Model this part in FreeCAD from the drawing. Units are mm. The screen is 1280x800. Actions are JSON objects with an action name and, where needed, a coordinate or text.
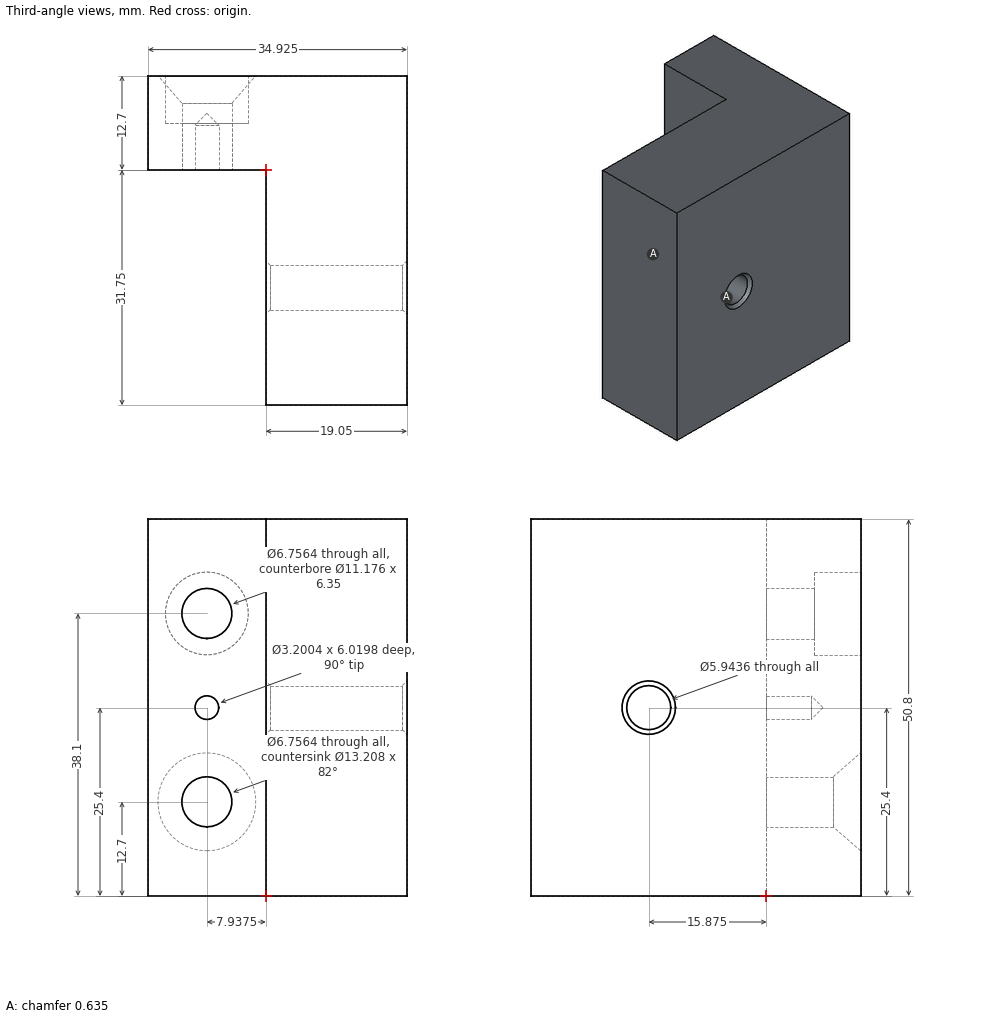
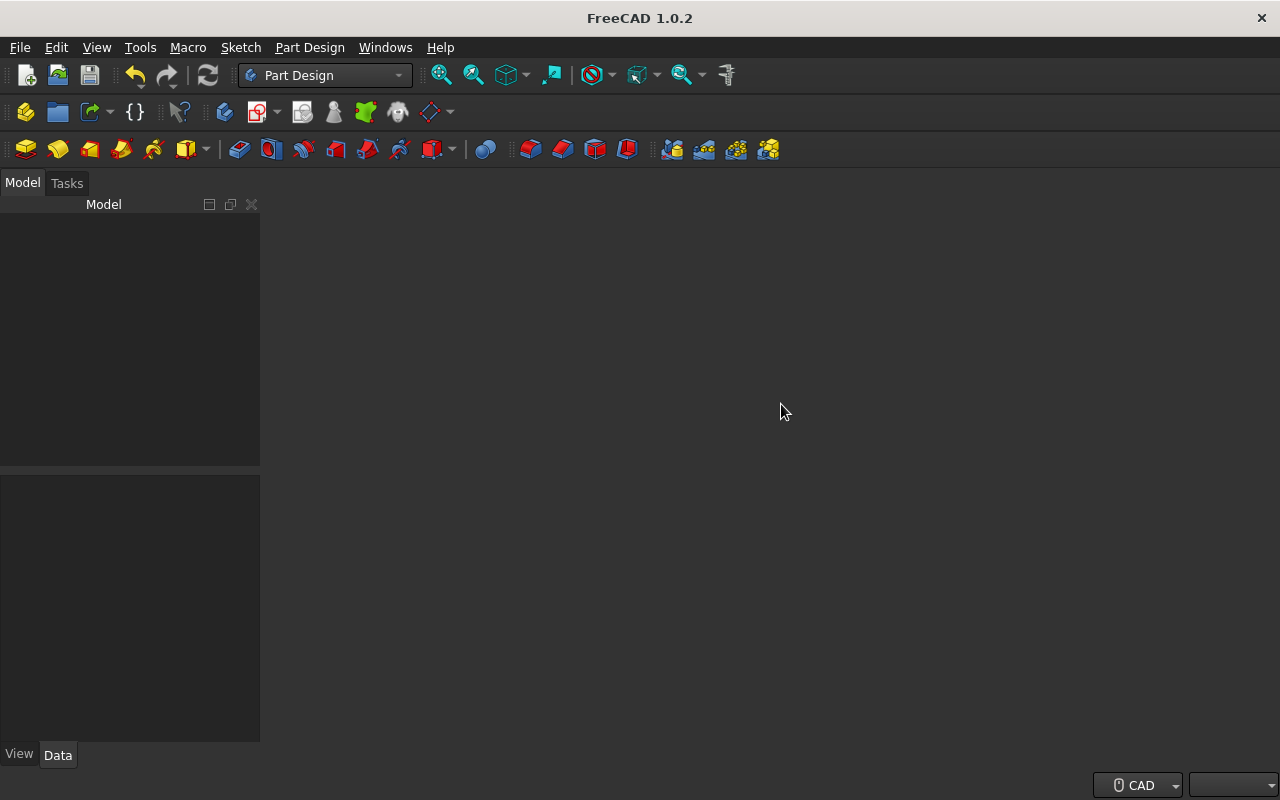
{"action": "left_click", "coordinate": [26, 76]}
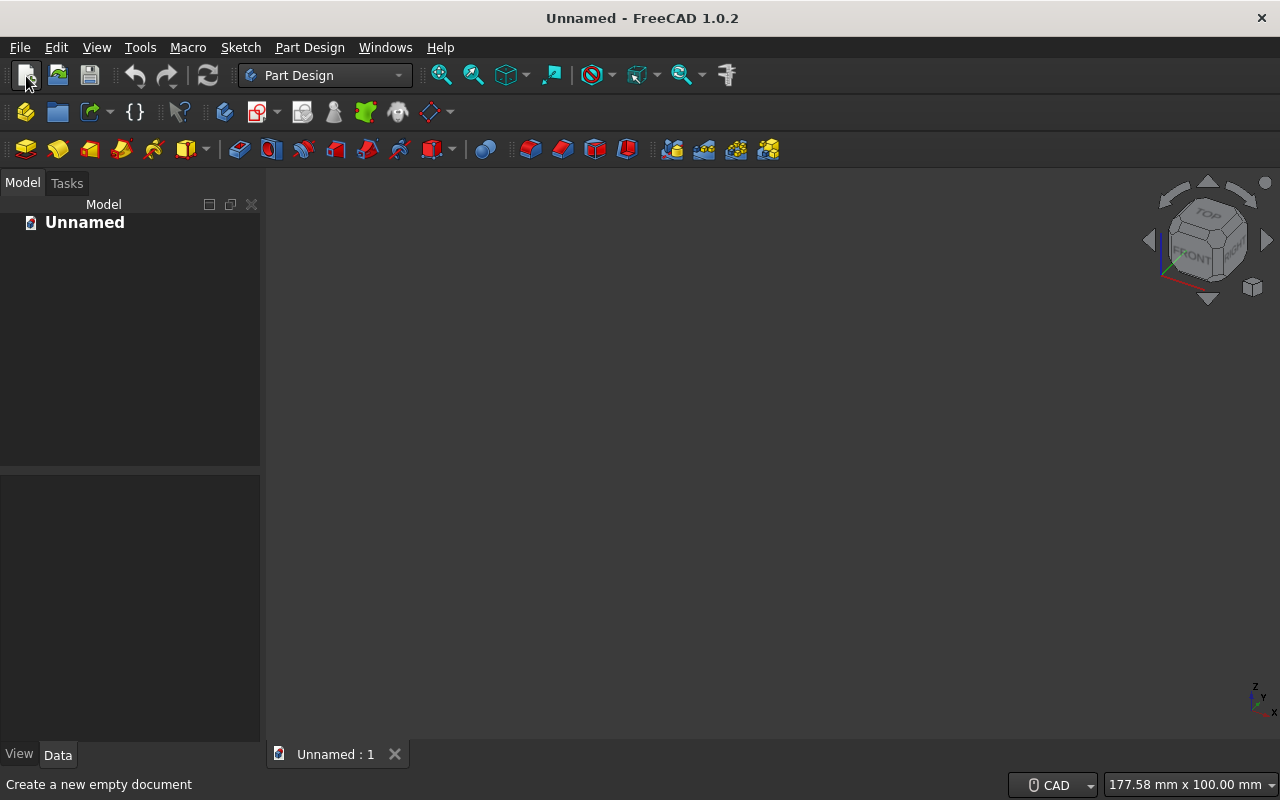
{"action": "left_click", "coordinate": [258, 112]}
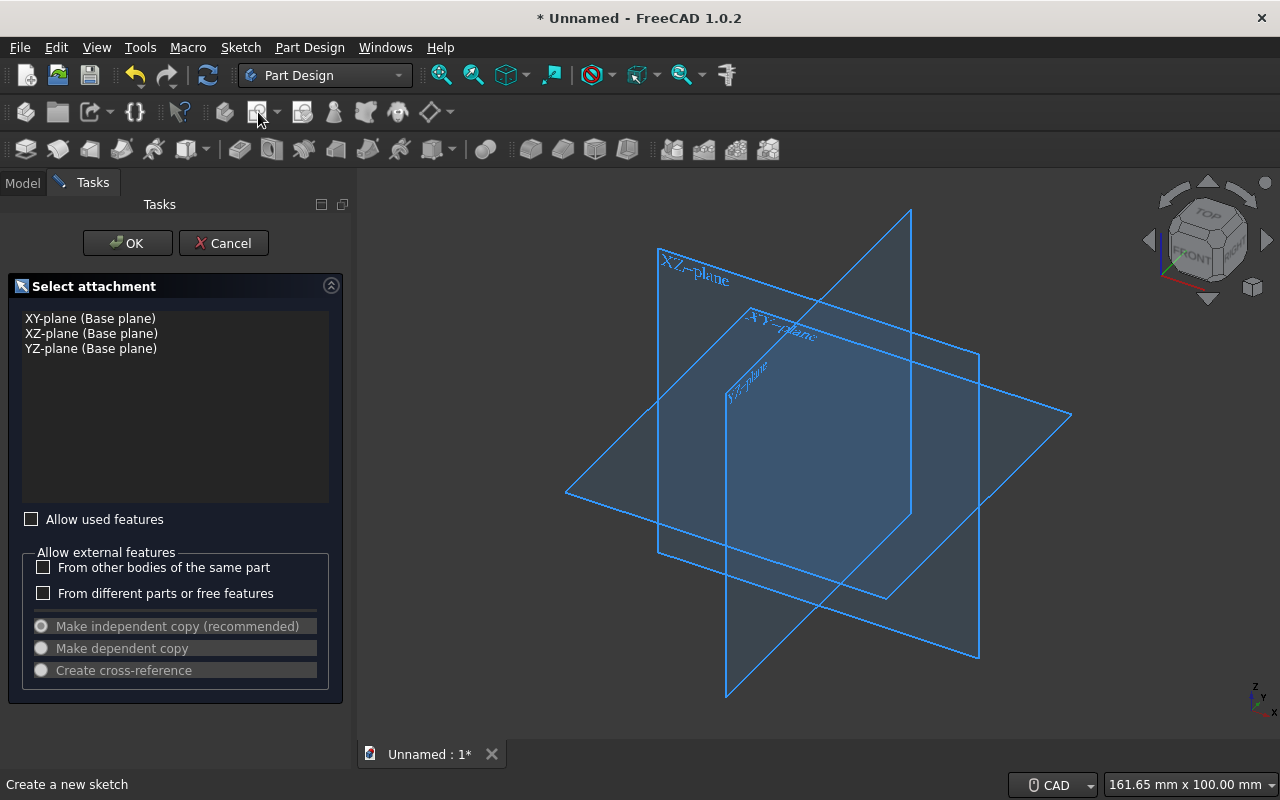
{"action": "left_click", "coordinate": [82, 318]}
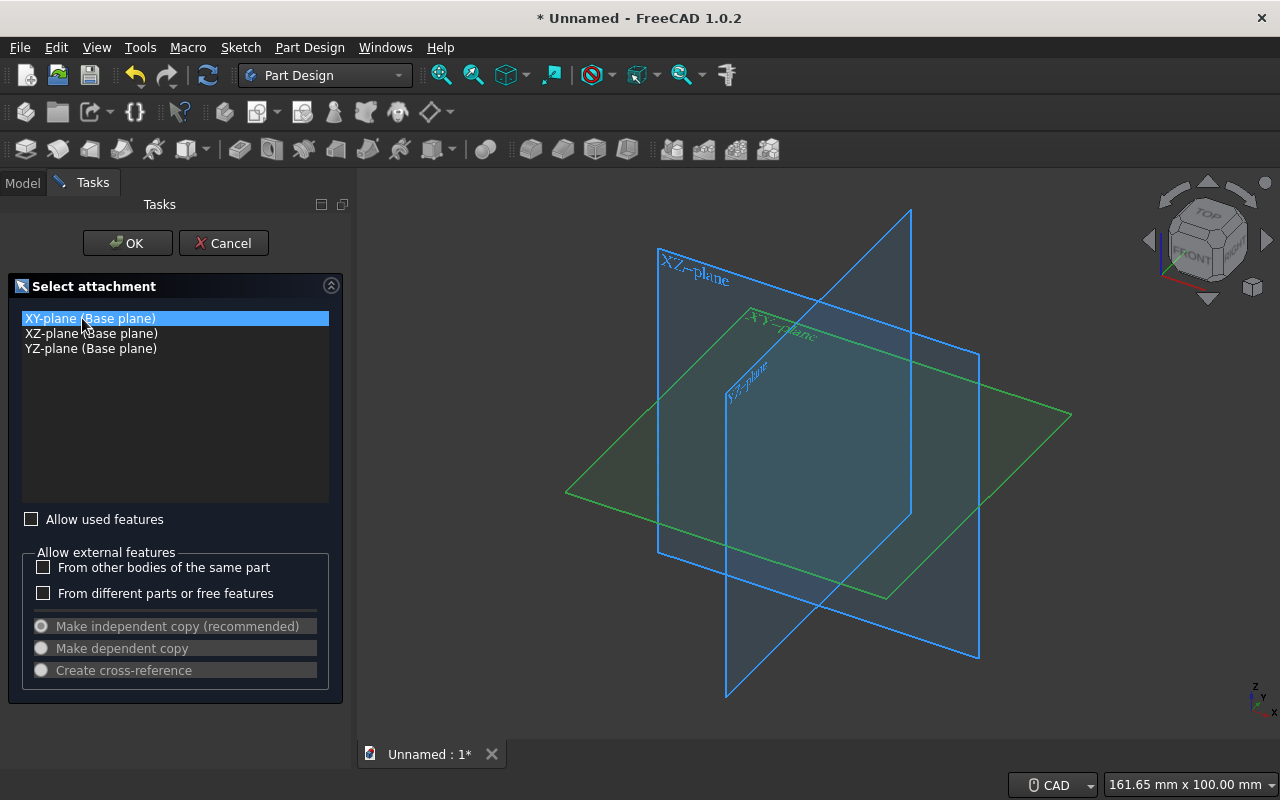
{"action": "left_click", "coordinate": [128, 243]}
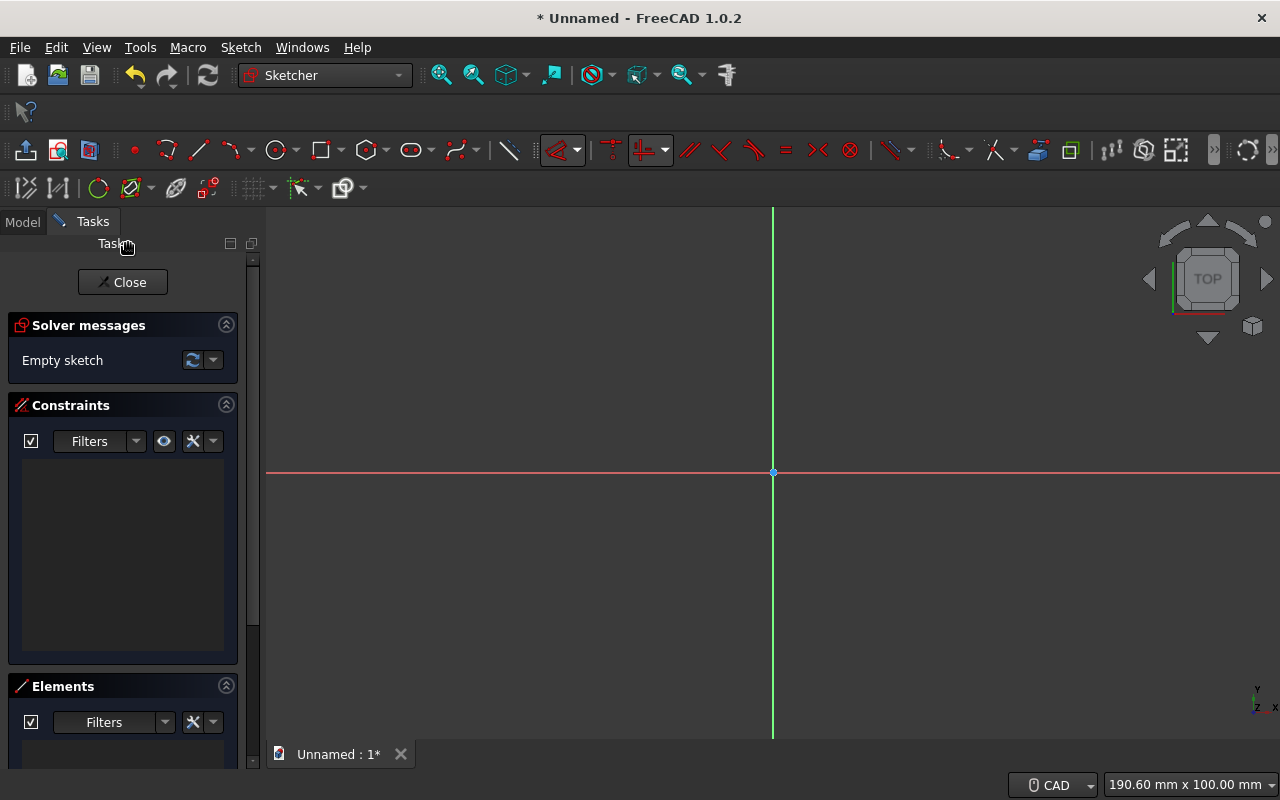
{"action": "scroll", "coordinate": [938, 627], "scroll_direction": "up", "scroll_amount": 2}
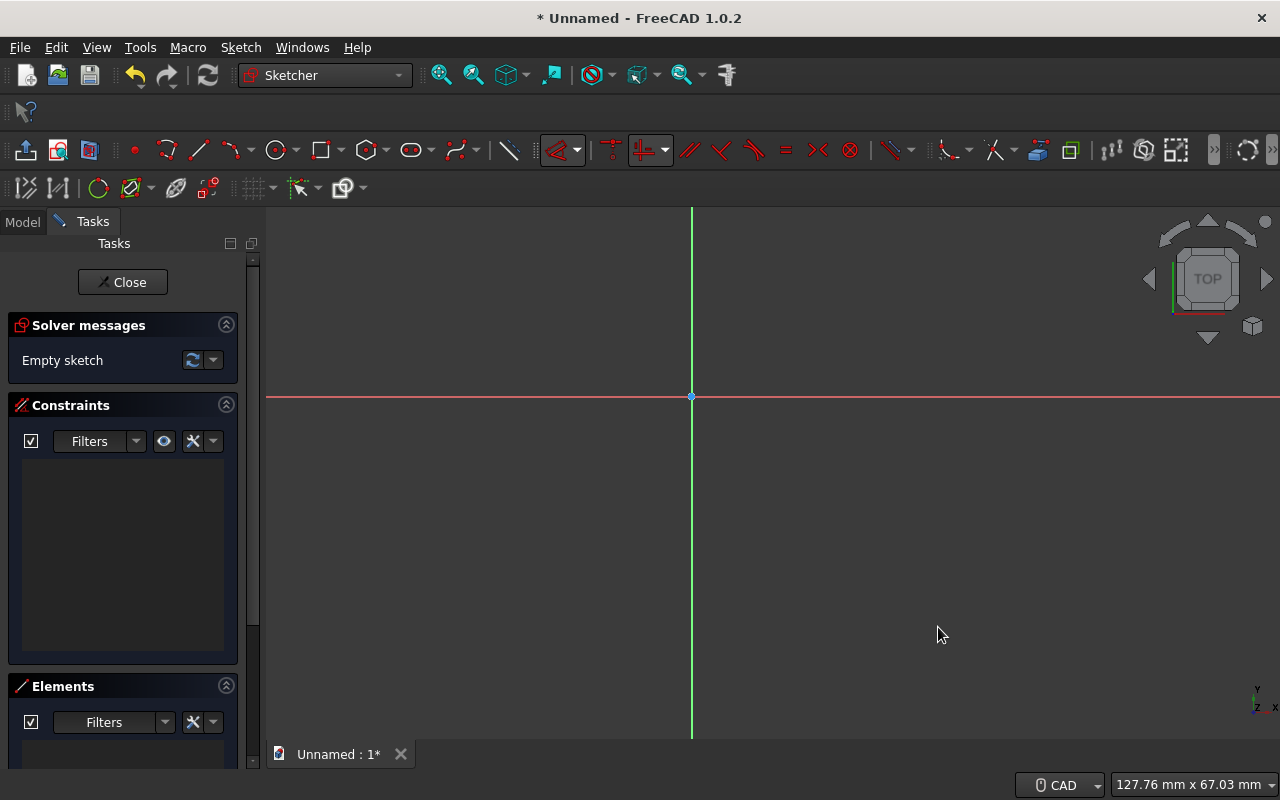
{"action": "left_click", "coordinate": [168, 150]}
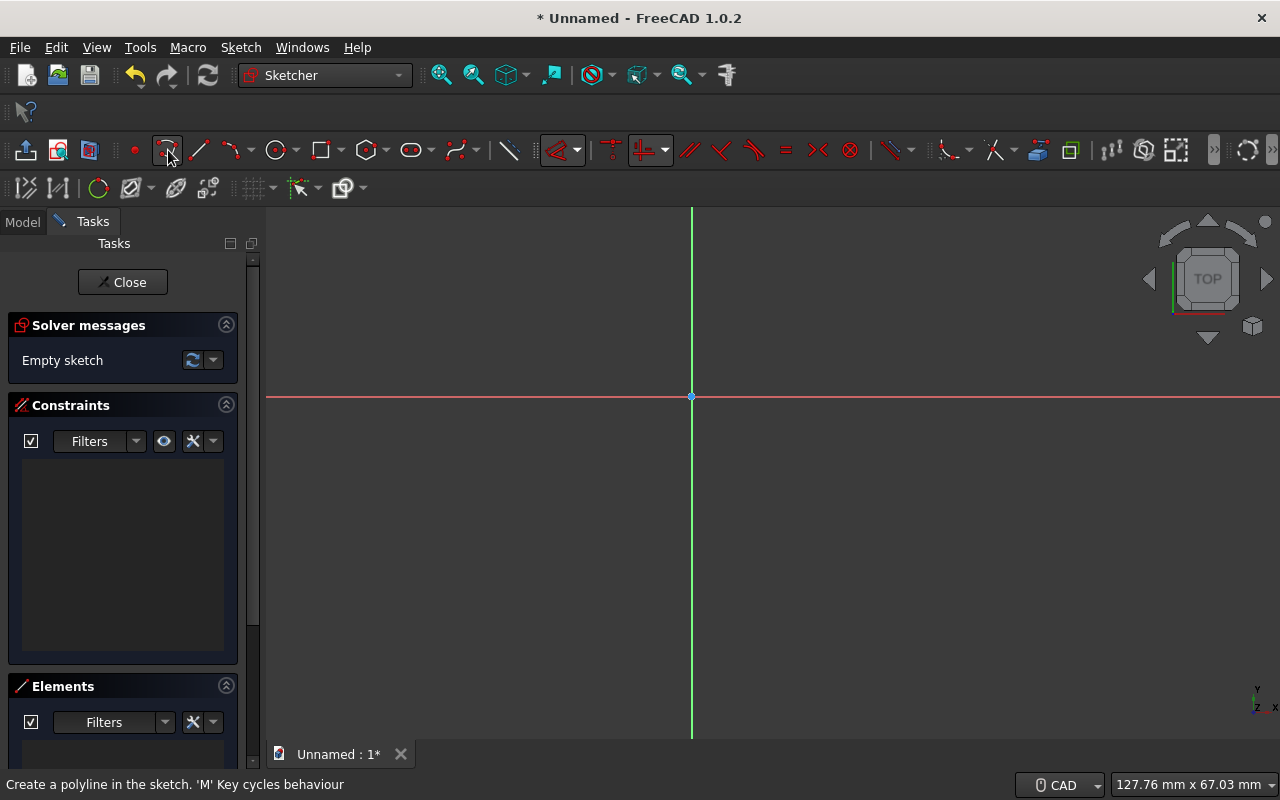
{"action": "left_click", "coordinate": [692, 397]}
{"action": "left_click", "coordinate": [701, 649]}
{"action": "left_click", "coordinate": [843, 649]}
{"action": "left_click", "coordinate": [843, 296]}
{"action": "left_click", "coordinate": [566, 296]}
{"action": "left_click", "coordinate": [566, 406]}
{"action": "left_click", "coordinate": [692, 397]}
{"action": "key", "text": "Escape"}
{"action": "key", "text": "Escape"}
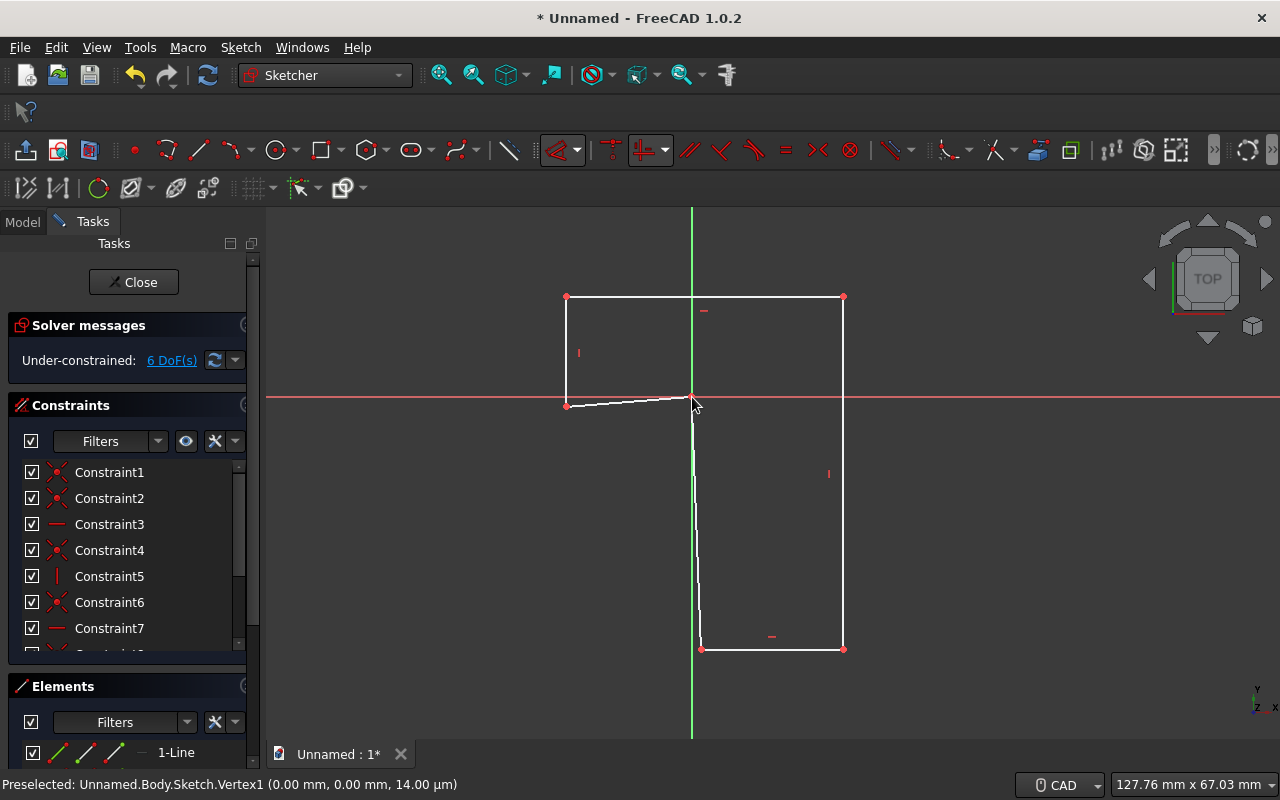
{"action": "left_click", "coordinate": [694, 473]}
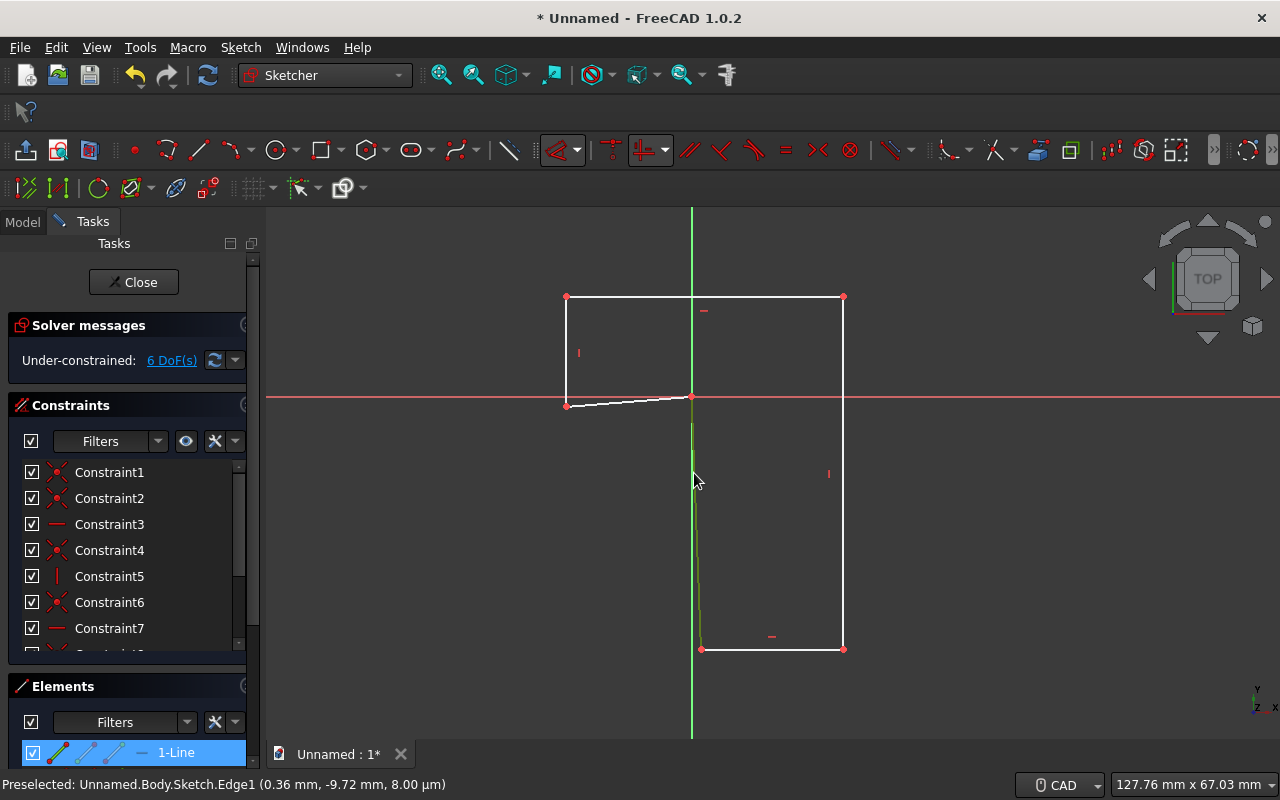
{"action": "left_click", "coordinate": [668, 150]}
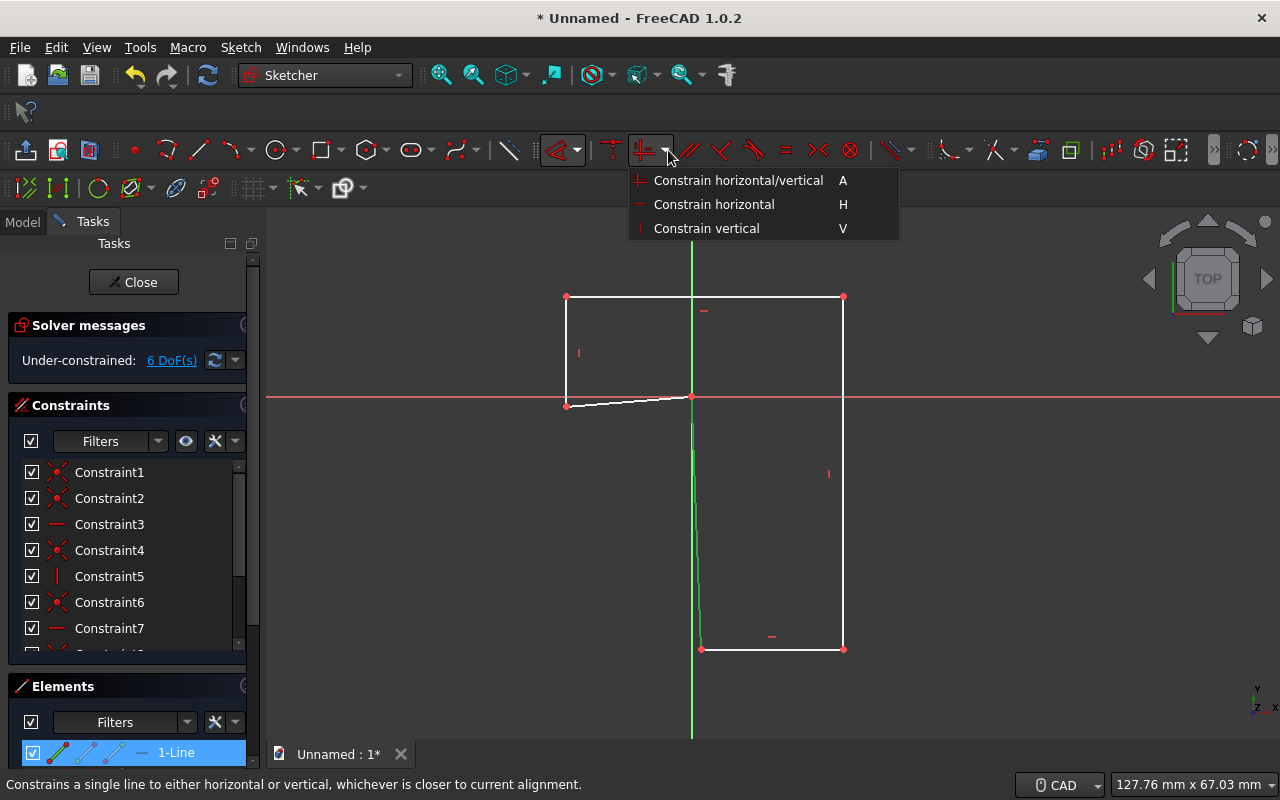
{"action": "left_click", "coordinate": [764, 228]}